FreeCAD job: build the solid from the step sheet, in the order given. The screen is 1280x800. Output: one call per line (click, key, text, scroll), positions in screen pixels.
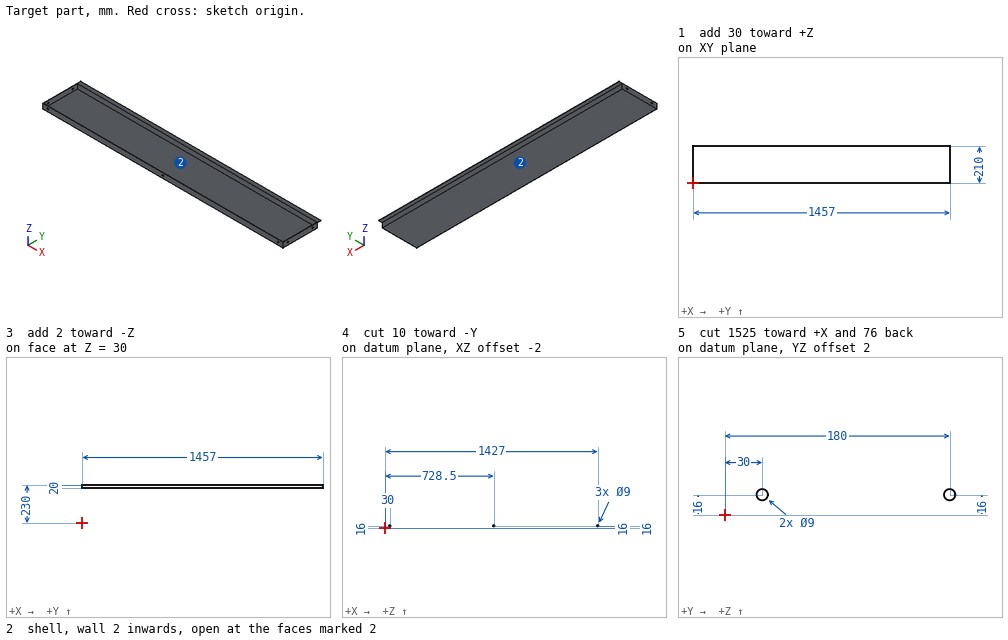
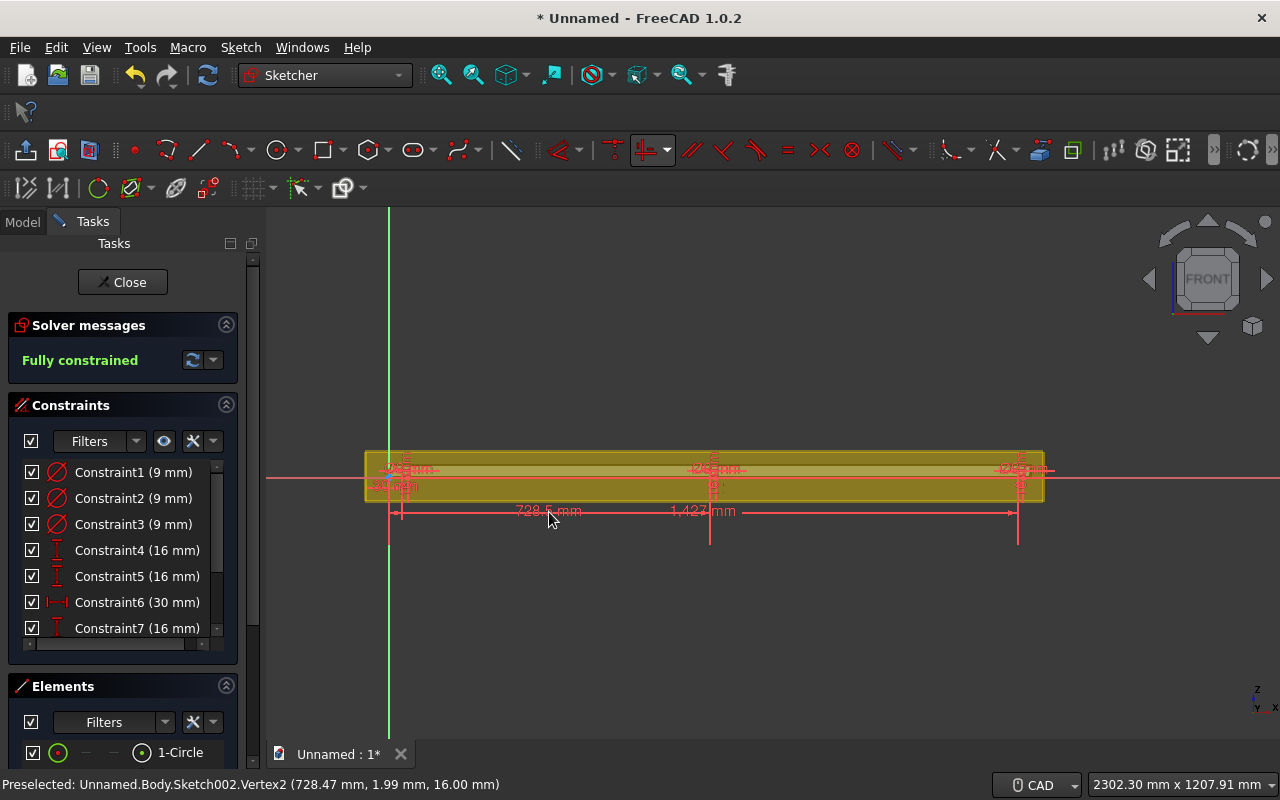
click(123, 282)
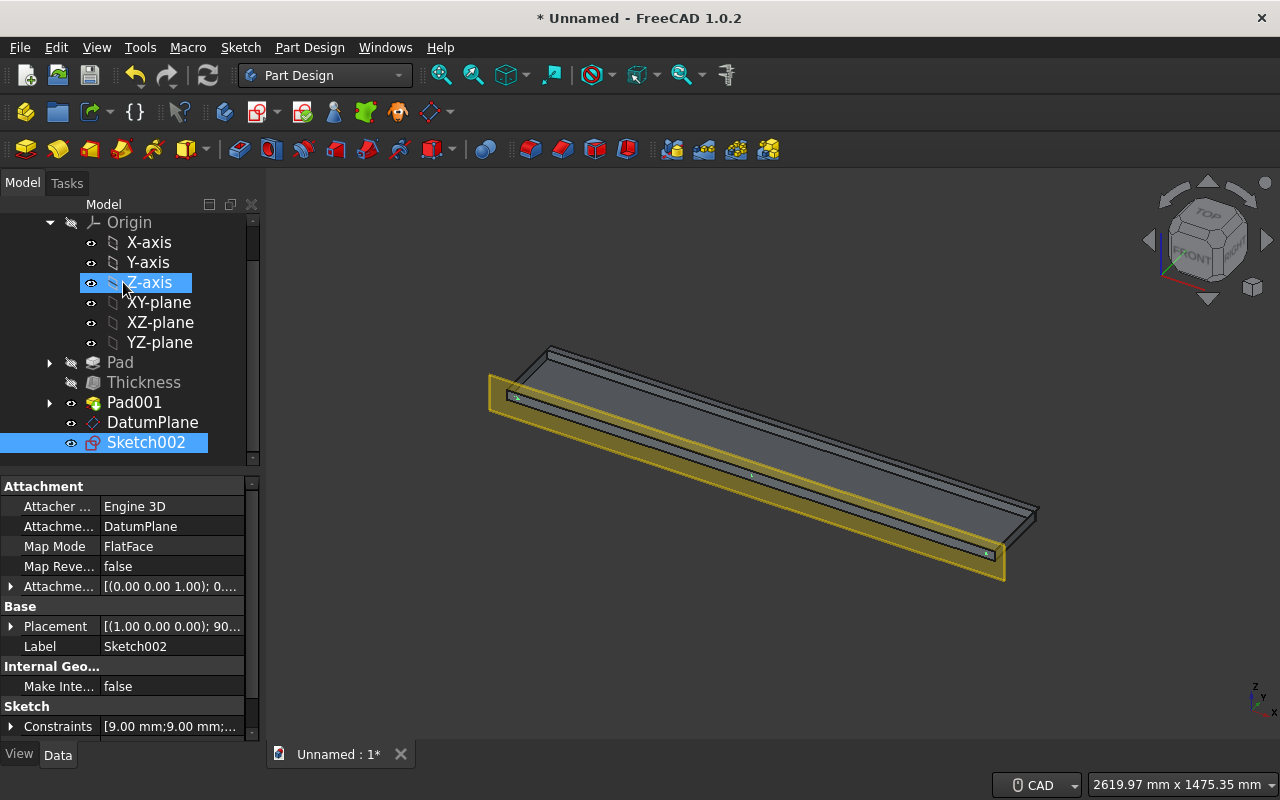
click(240, 150)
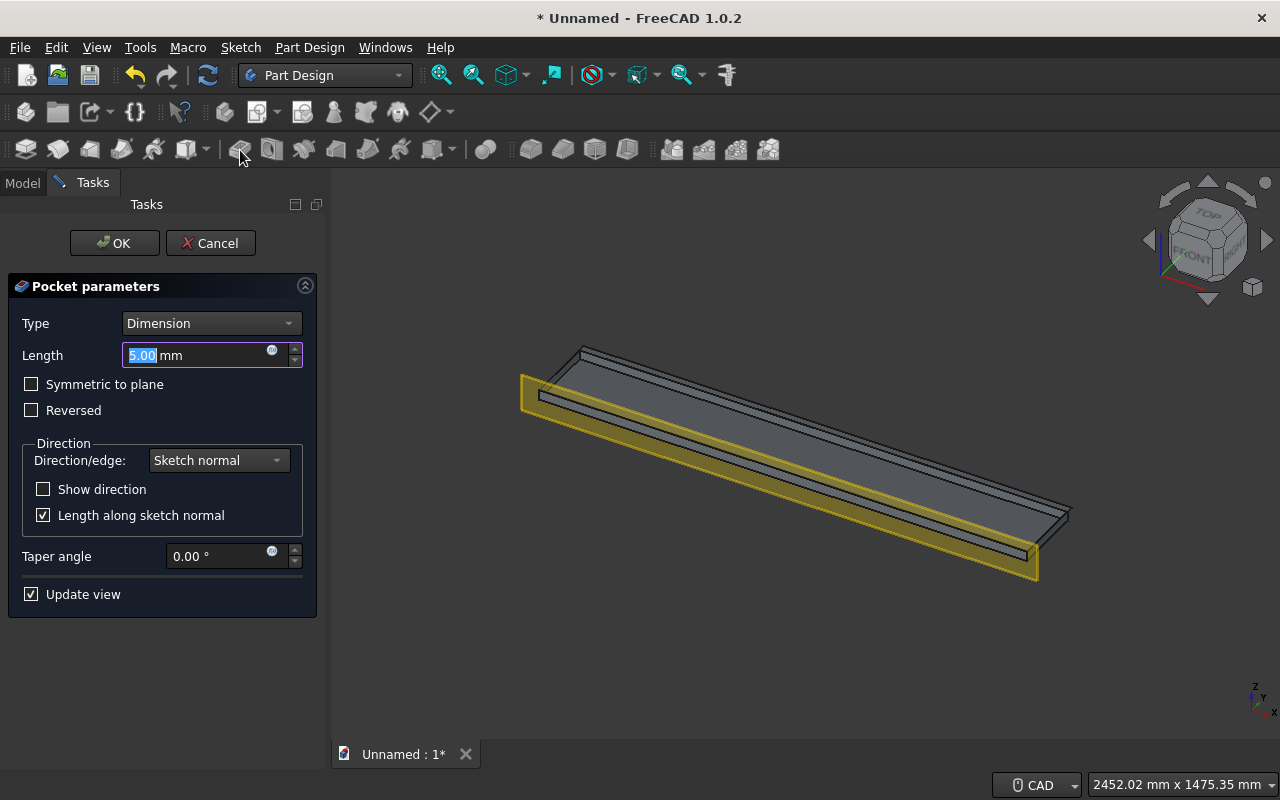
text(10)
key(Tab)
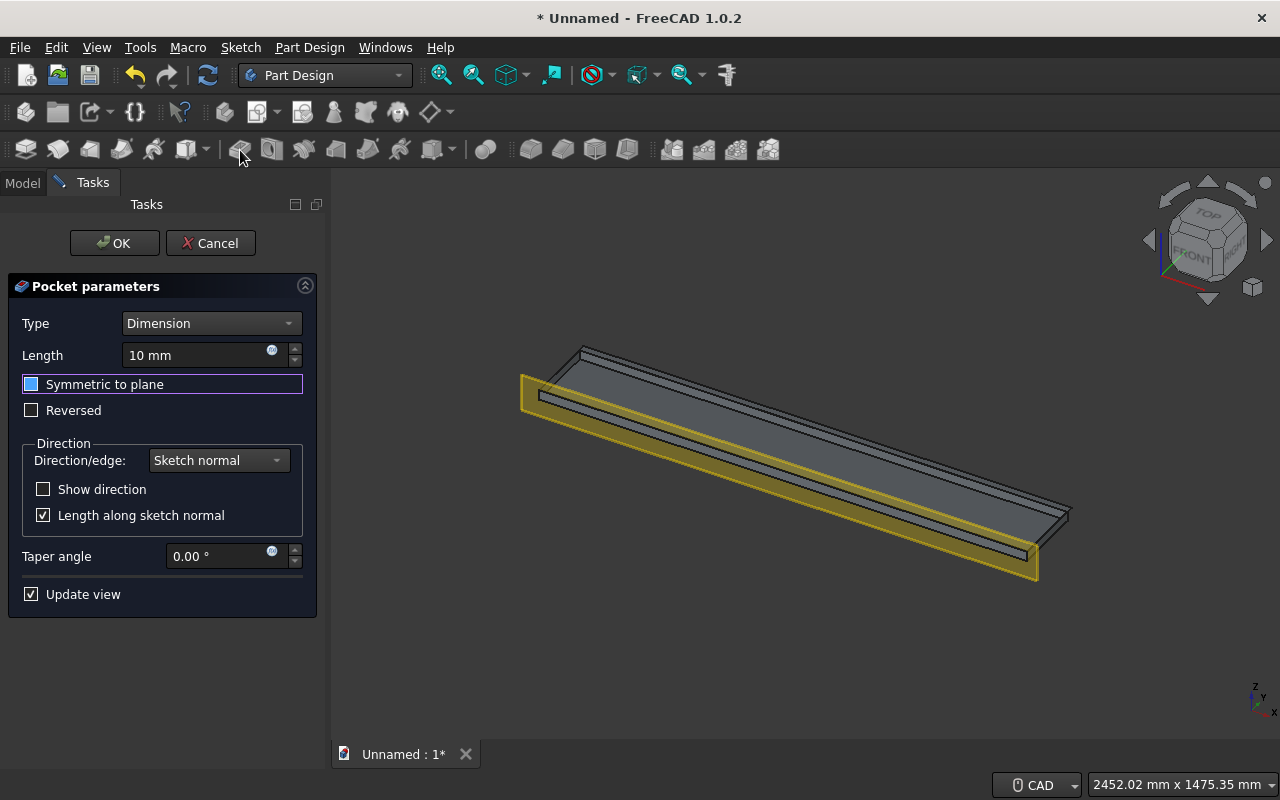
click(30, 410)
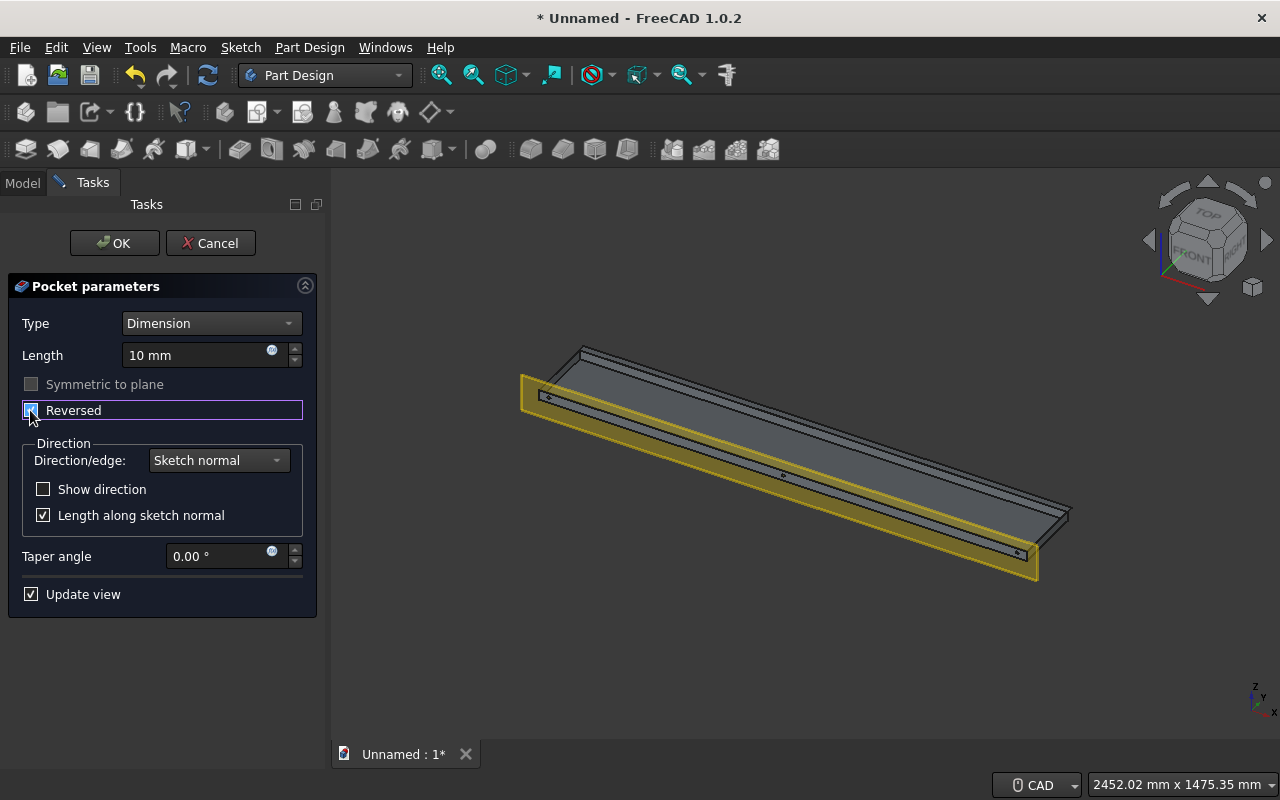
click(115, 243)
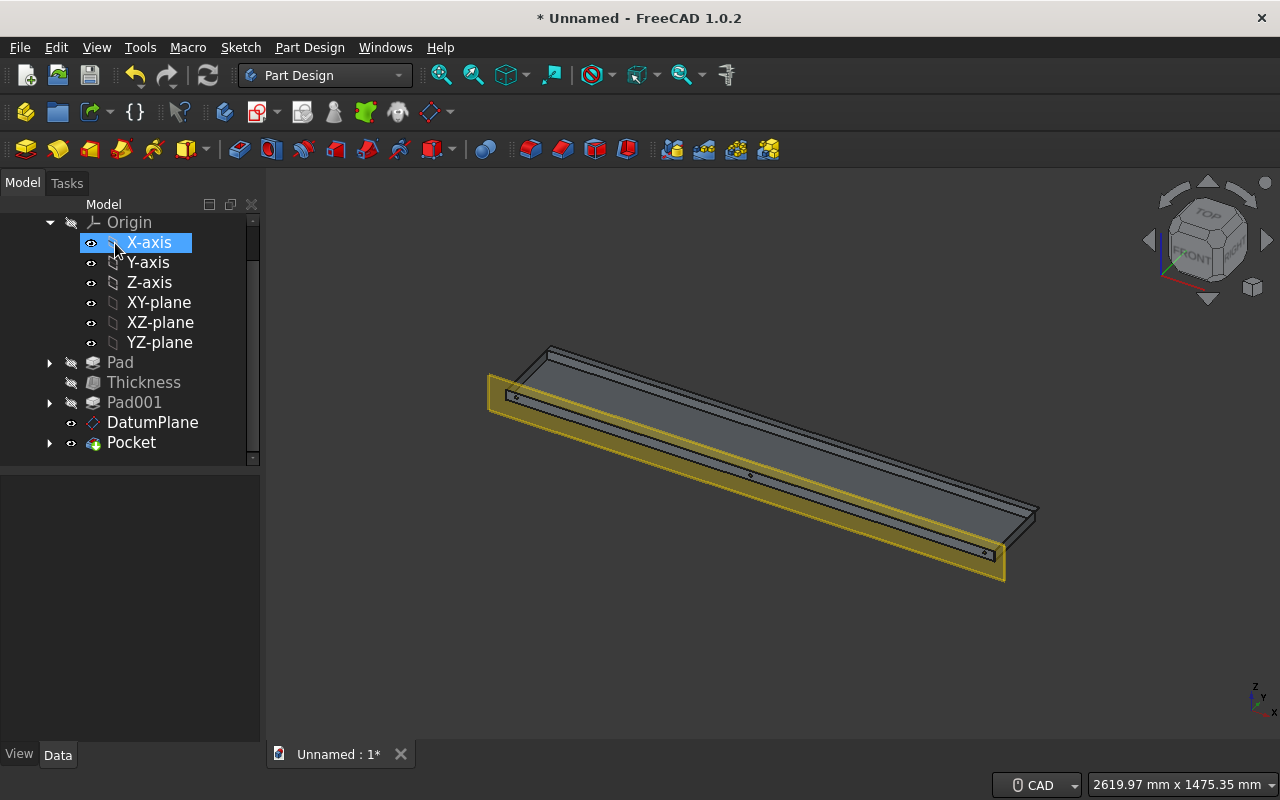
click(116, 423)
key(space)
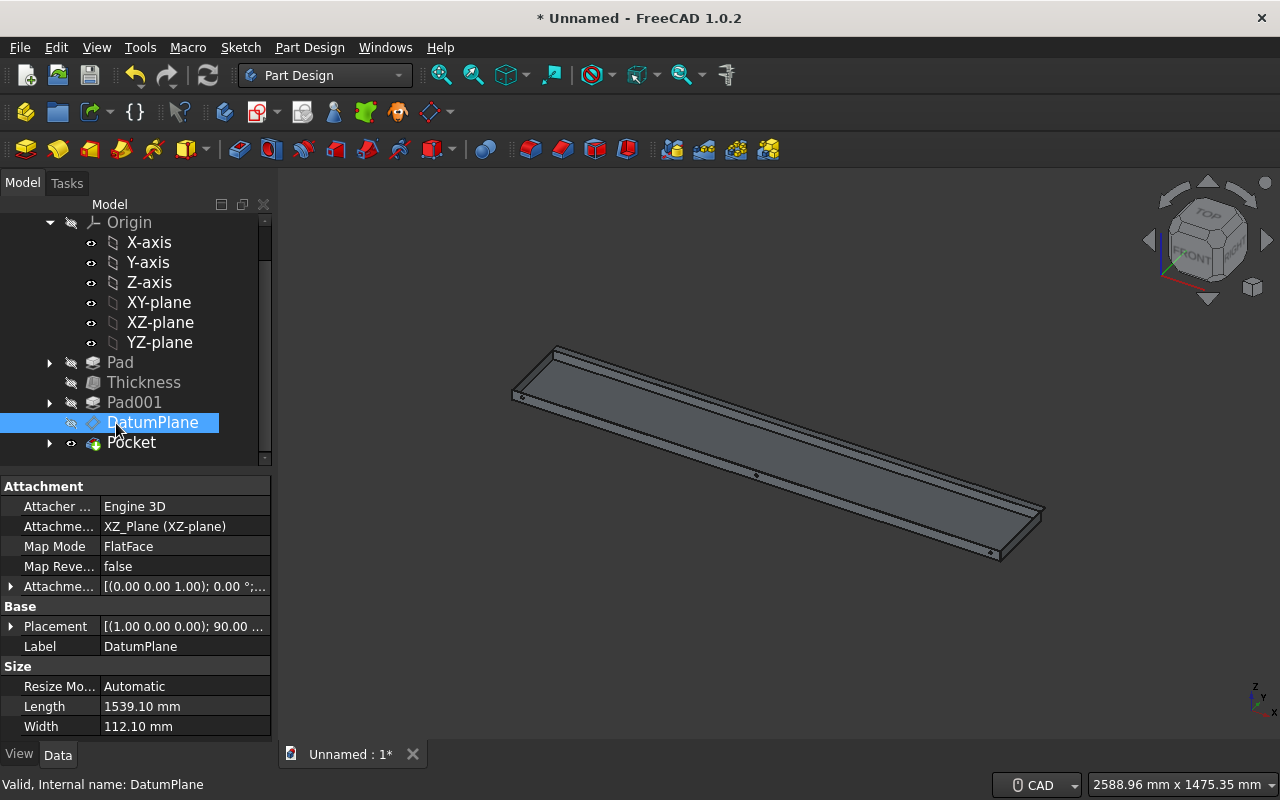
click(136, 343)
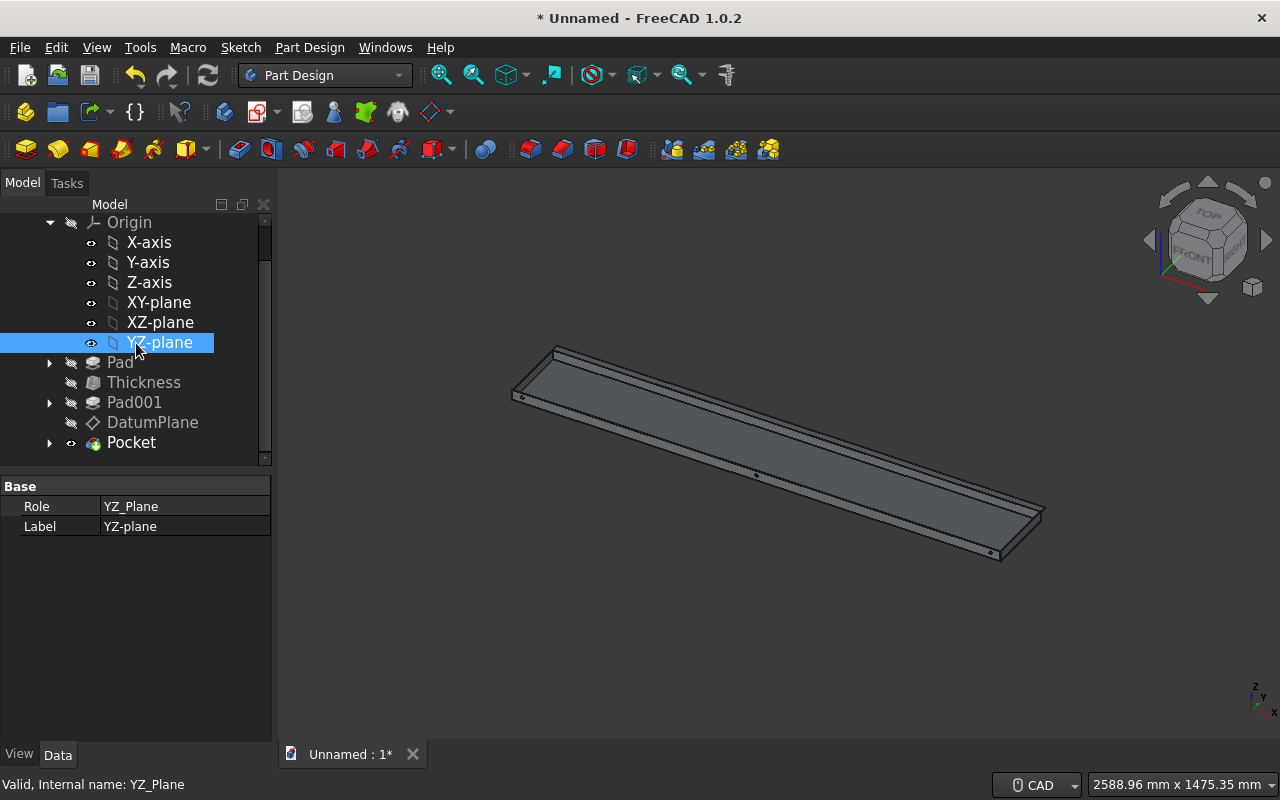
click(430, 112)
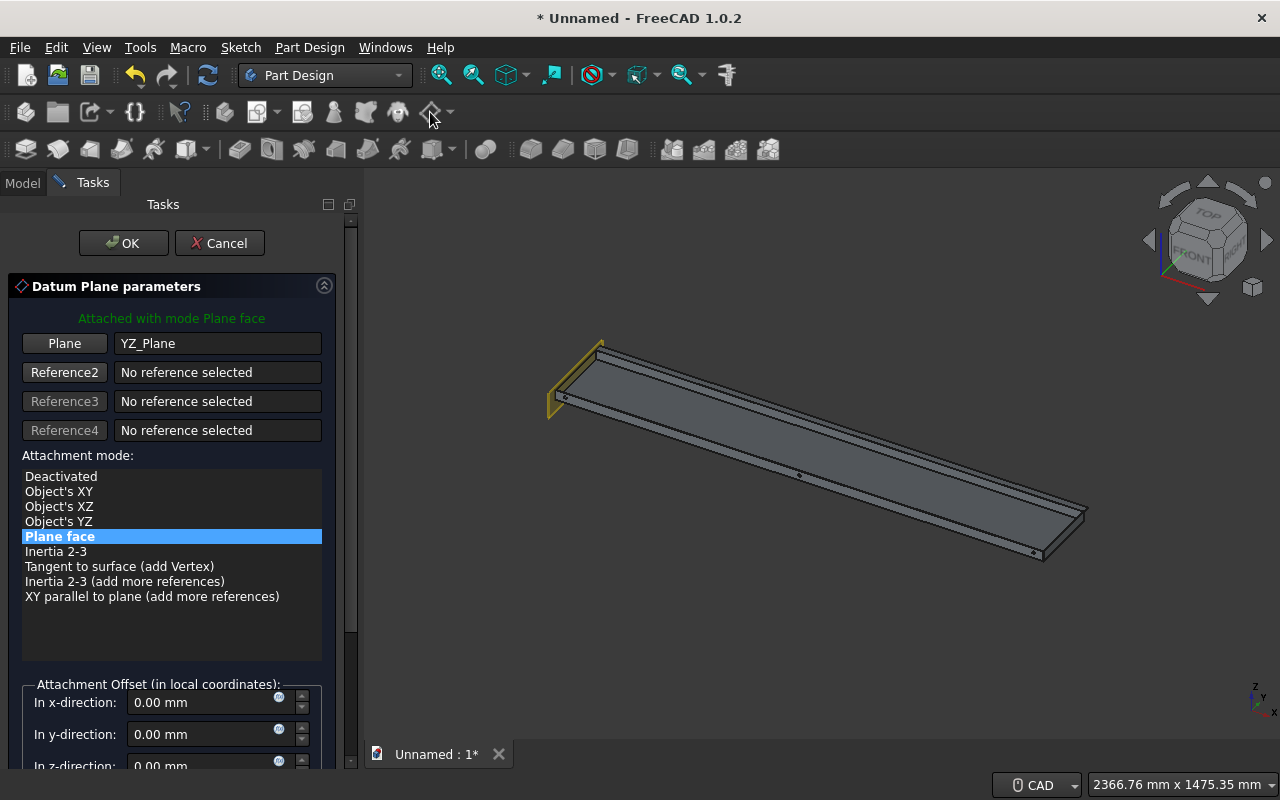
scroll(351, 491, down, 2)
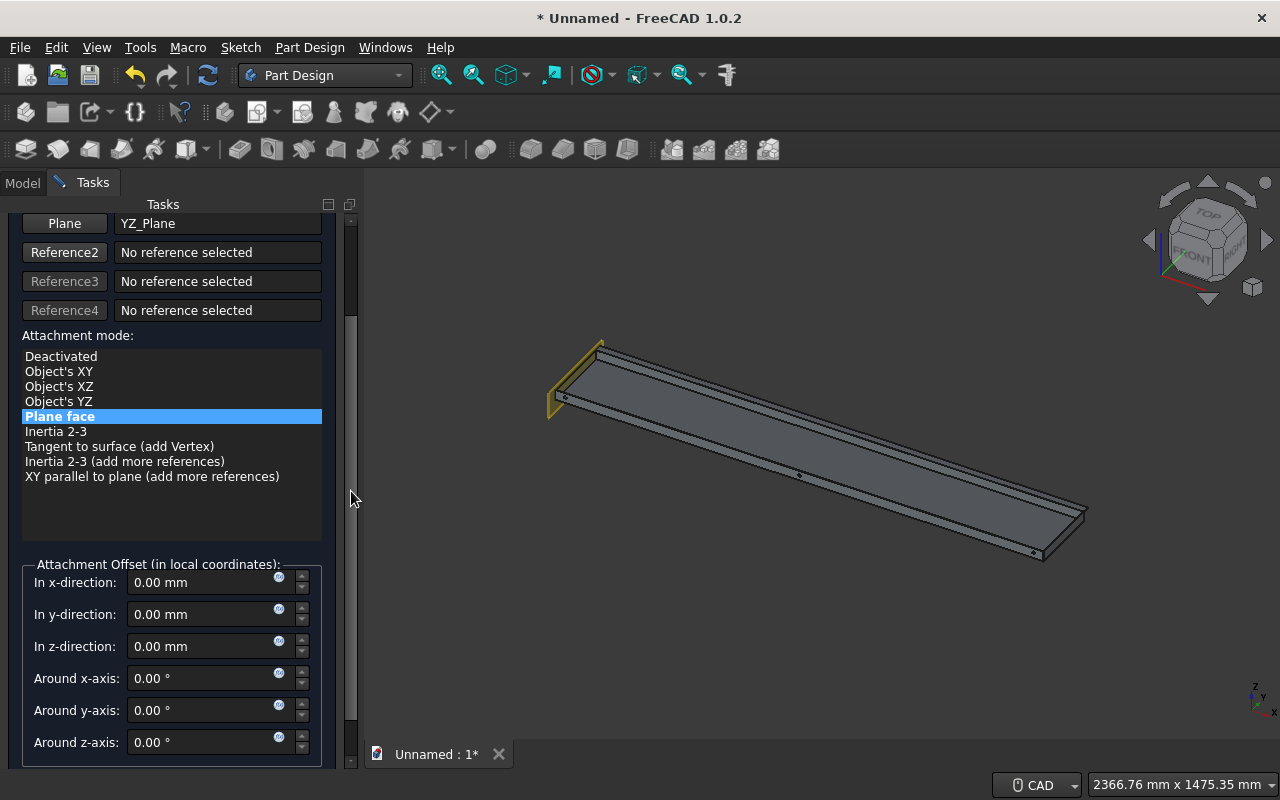
triple_click(210, 646)